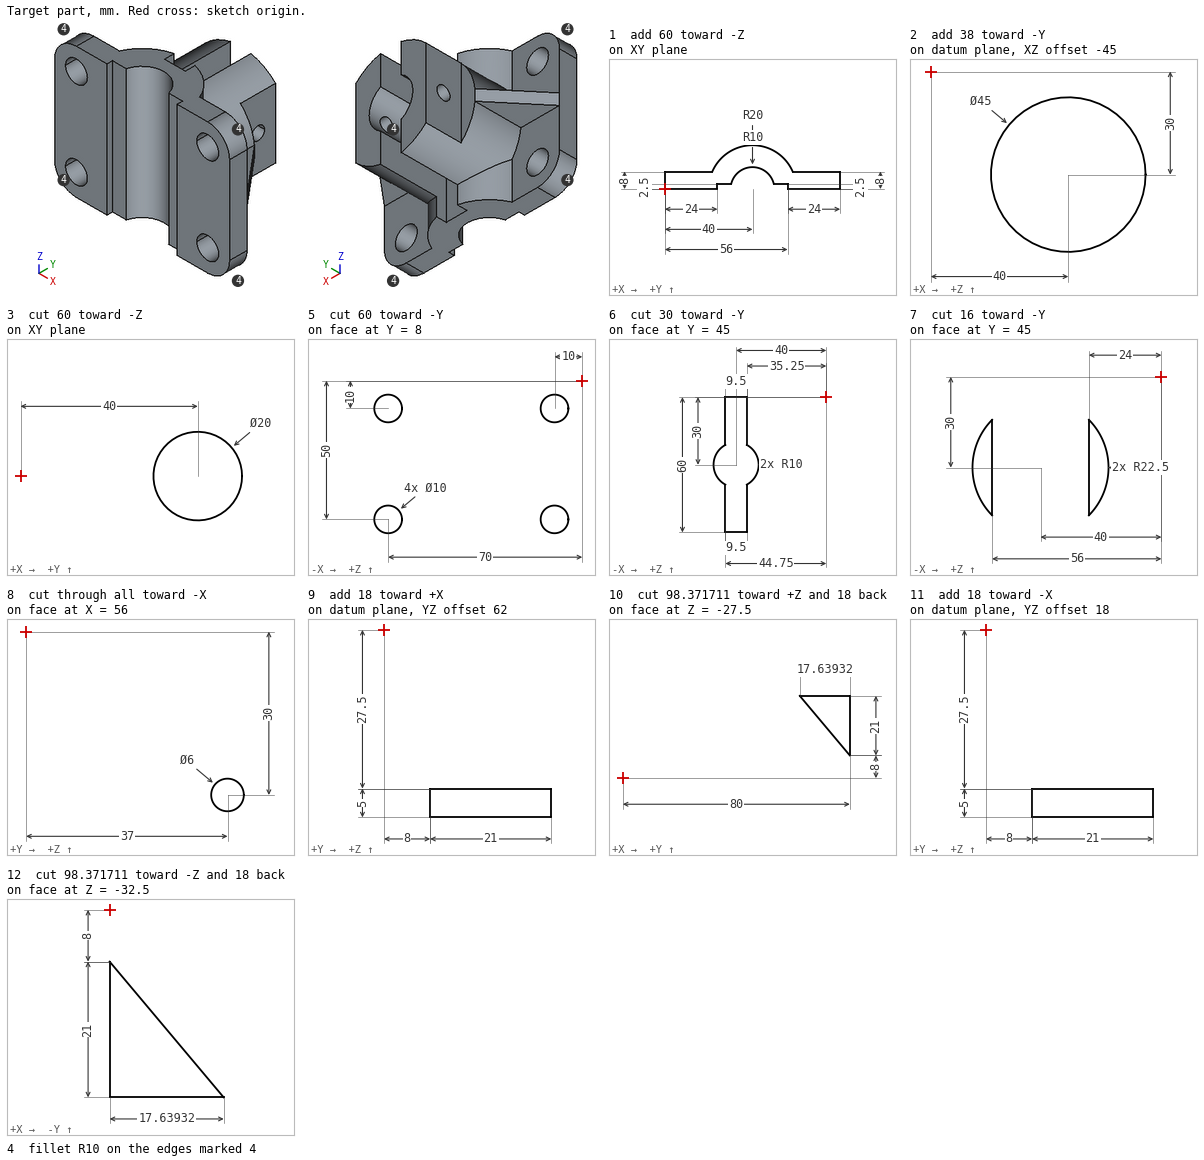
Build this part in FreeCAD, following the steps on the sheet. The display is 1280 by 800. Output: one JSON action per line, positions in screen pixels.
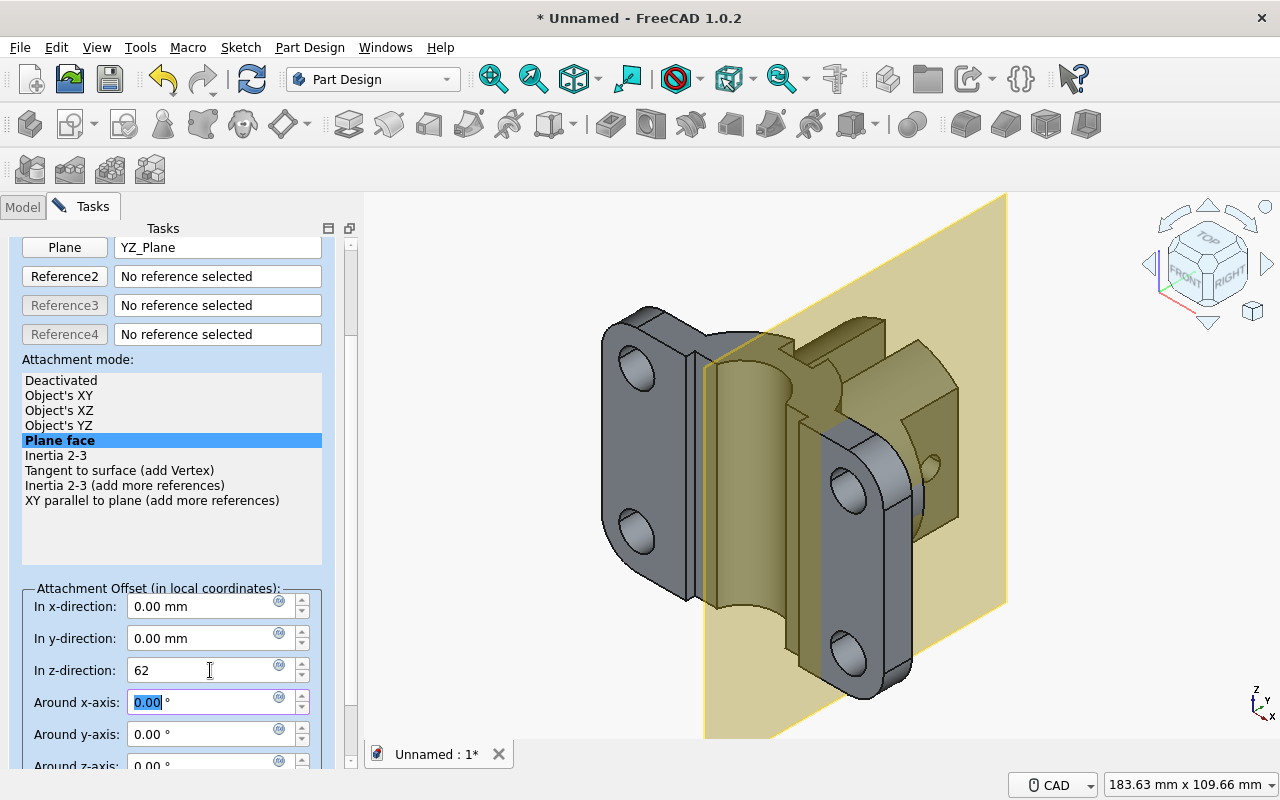
{"action": "scroll", "coordinate": [351, 503], "scroll_direction": "up", "scroll_amount": 3}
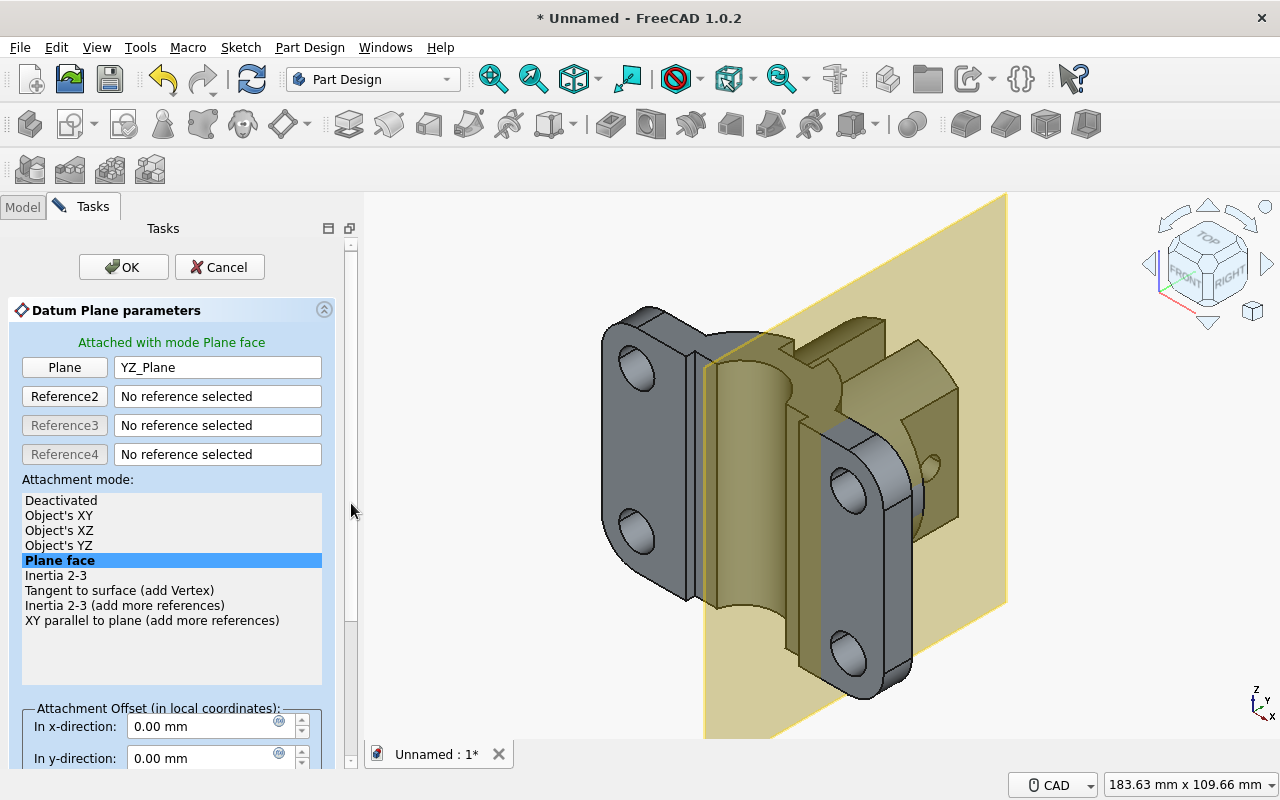
{"action": "left_click", "coordinate": [124, 267]}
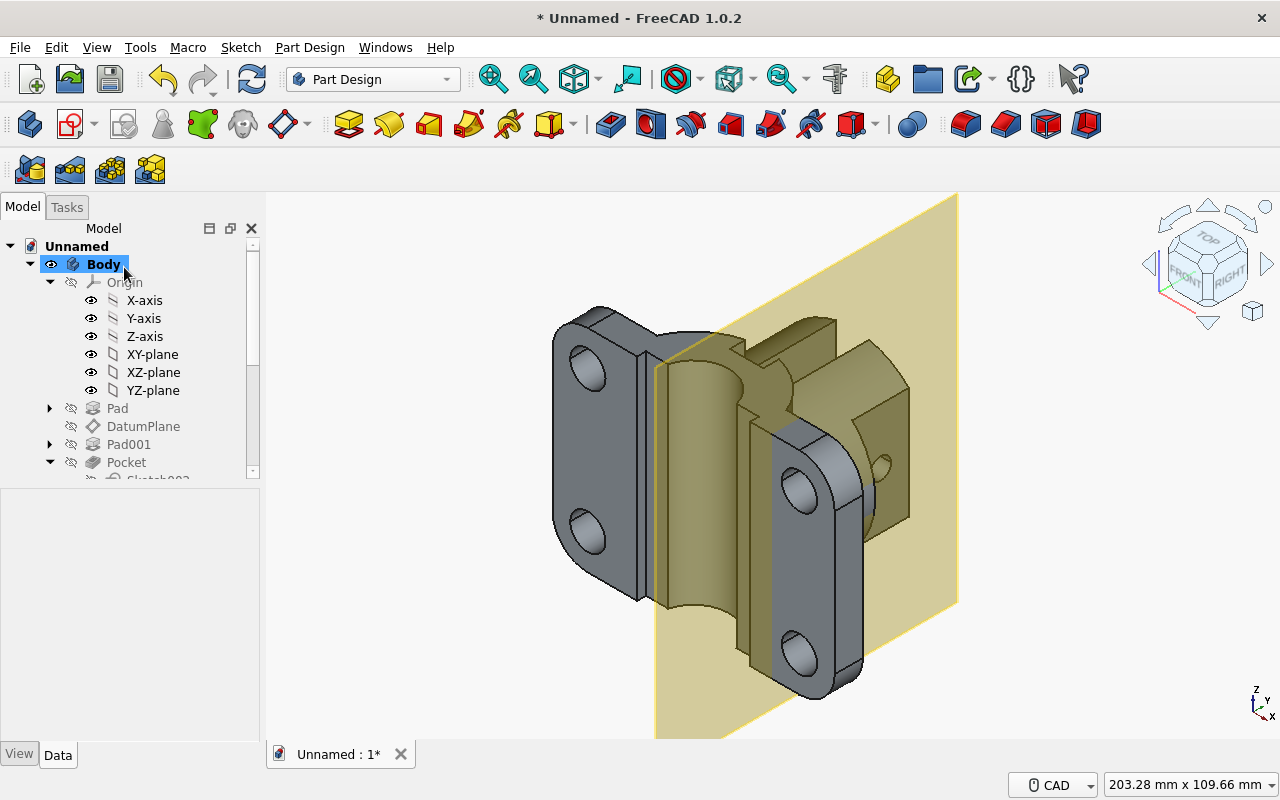
{"action": "scroll", "coordinate": [100, 350], "scroll_direction": "down", "scroll_amount": 3}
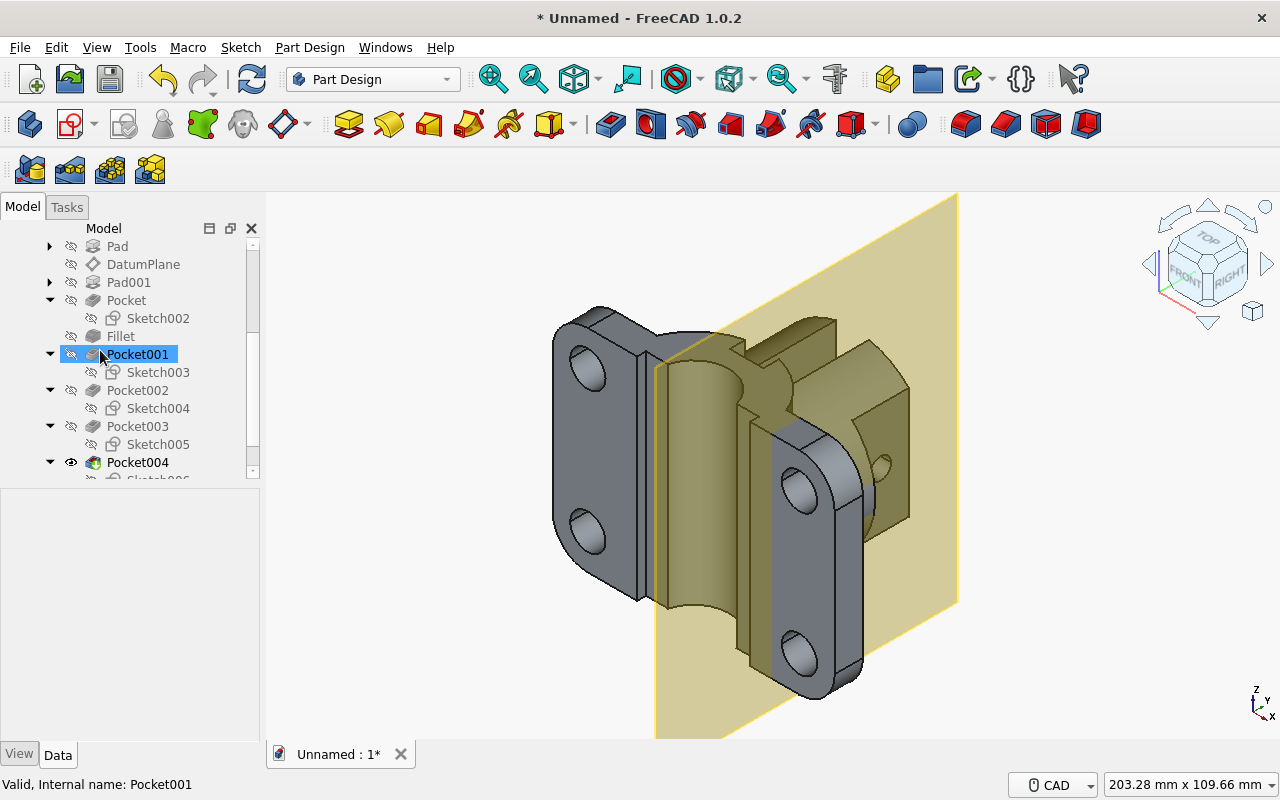
{"action": "scroll", "coordinate": [140, 350], "scroll_direction": "up", "scroll_amount": 15}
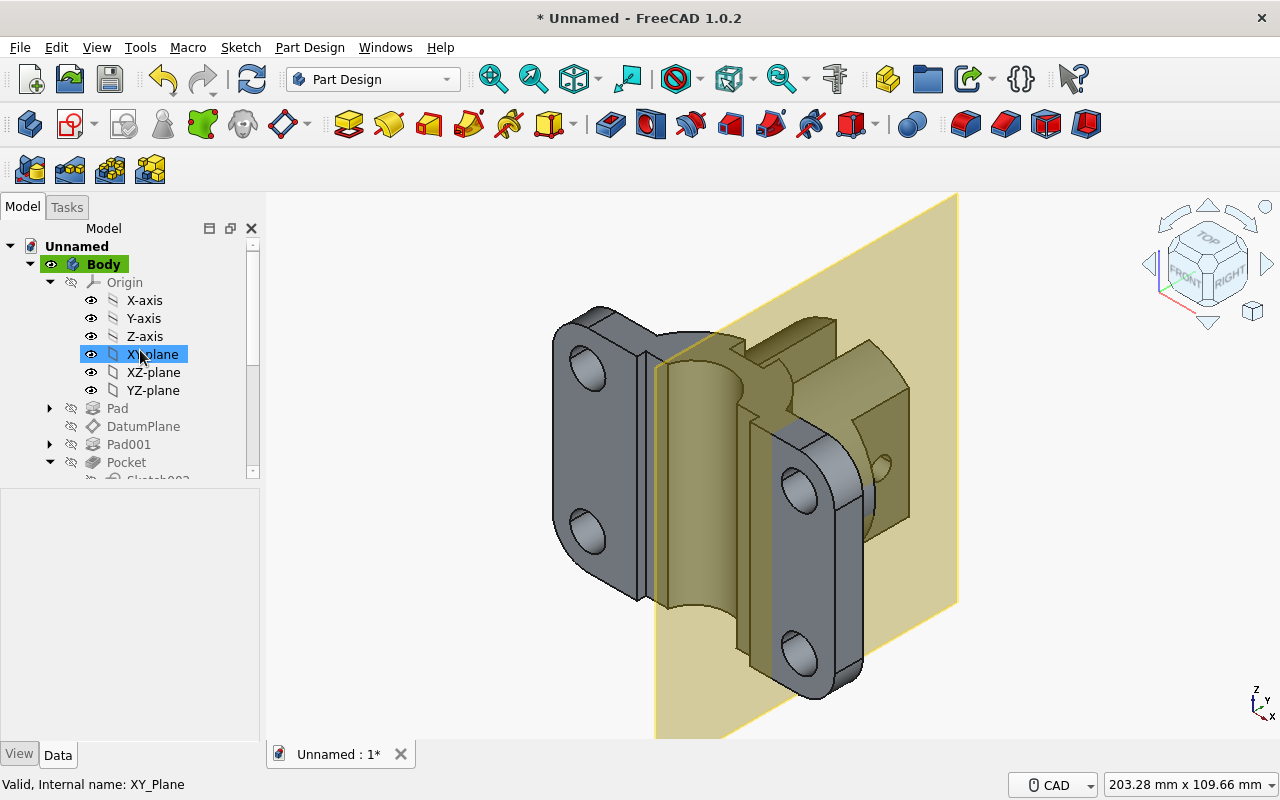
{"action": "scroll", "coordinate": [100, 350], "scroll_direction": "down", "scroll_amount": 6}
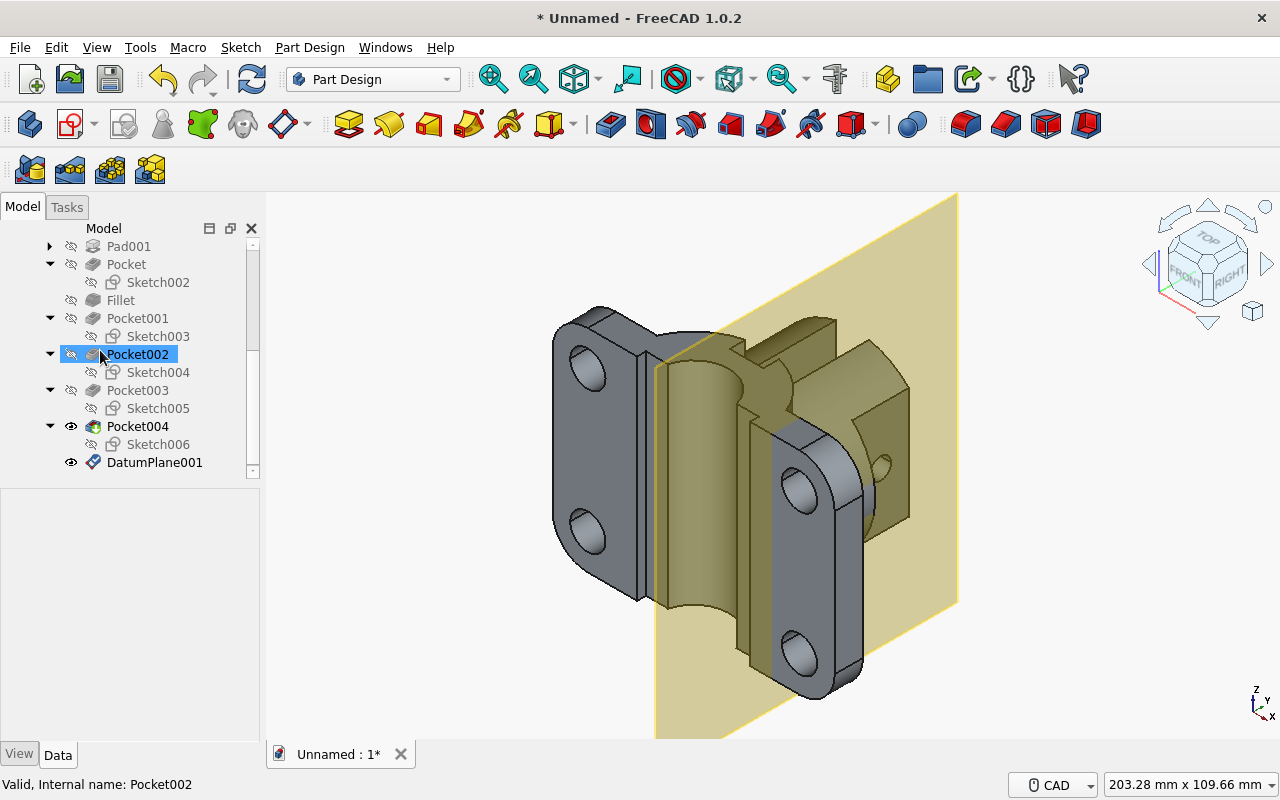
{"action": "left_click", "coordinate": [116, 462]}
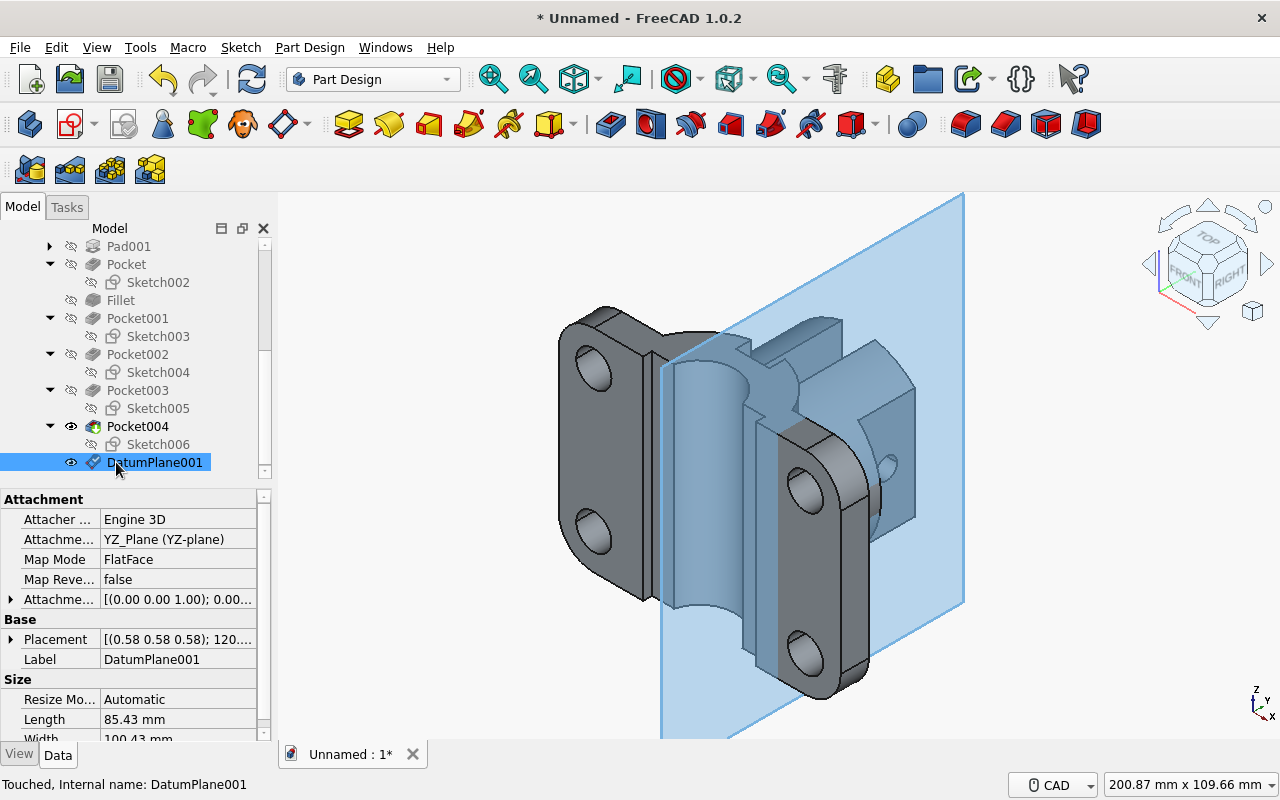
{"action": "left_click", "coordinate": [70, 124]}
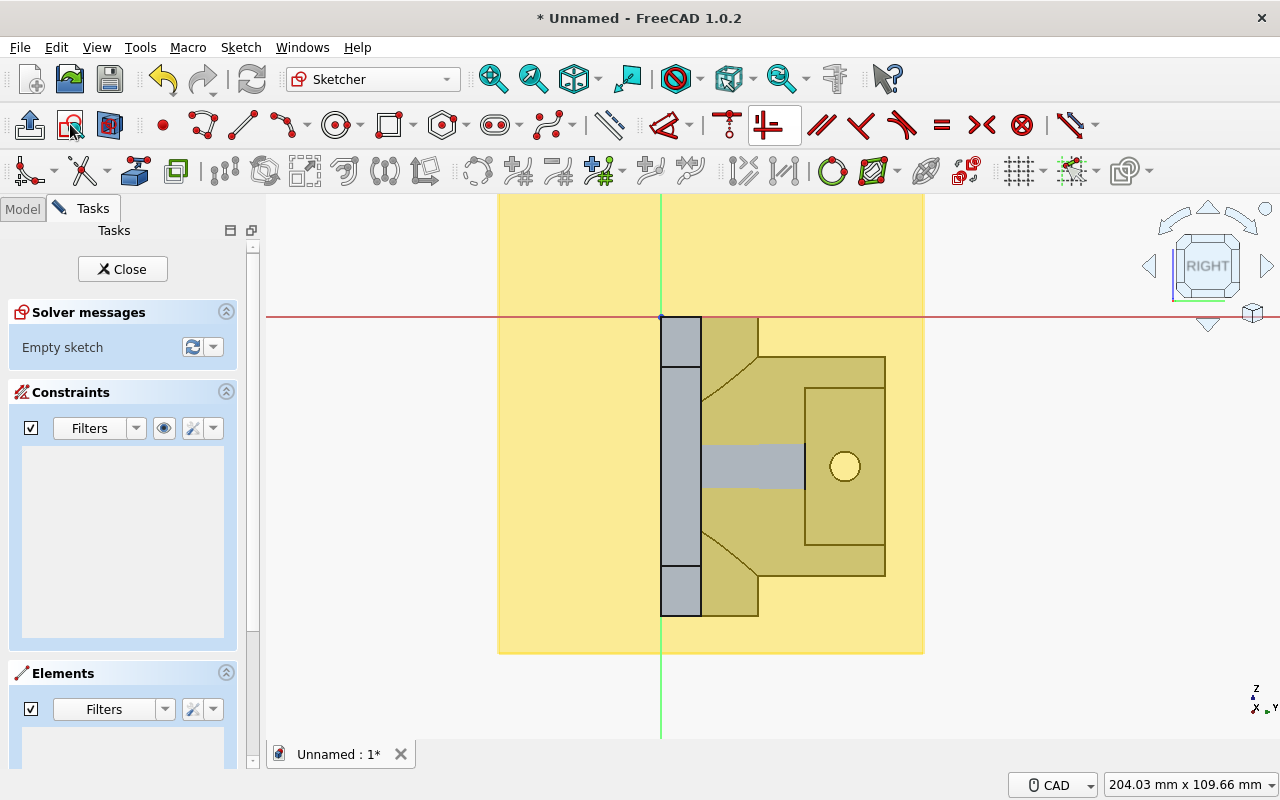
{"action": "left_click", "coordinate": [110, 126]}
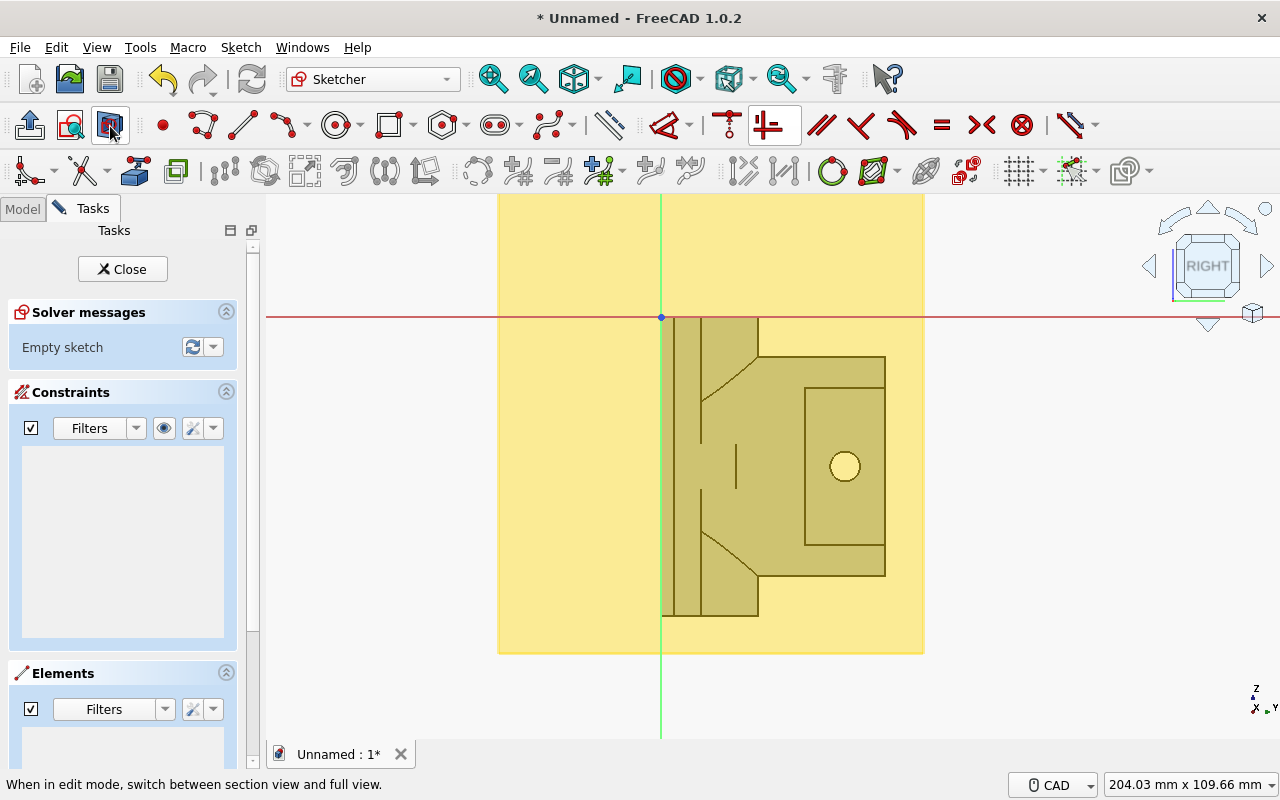
{"action": "scroll", "coordinate": [757, 342], "scroll_direction": "up", "scroll_amount": 4}